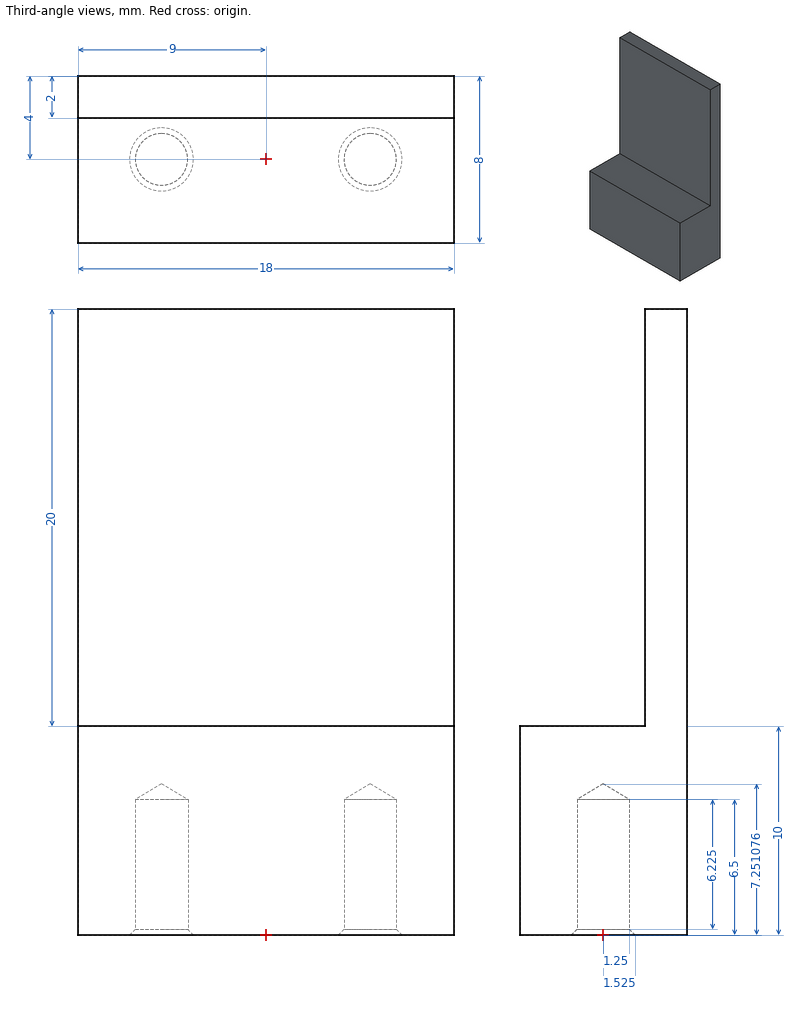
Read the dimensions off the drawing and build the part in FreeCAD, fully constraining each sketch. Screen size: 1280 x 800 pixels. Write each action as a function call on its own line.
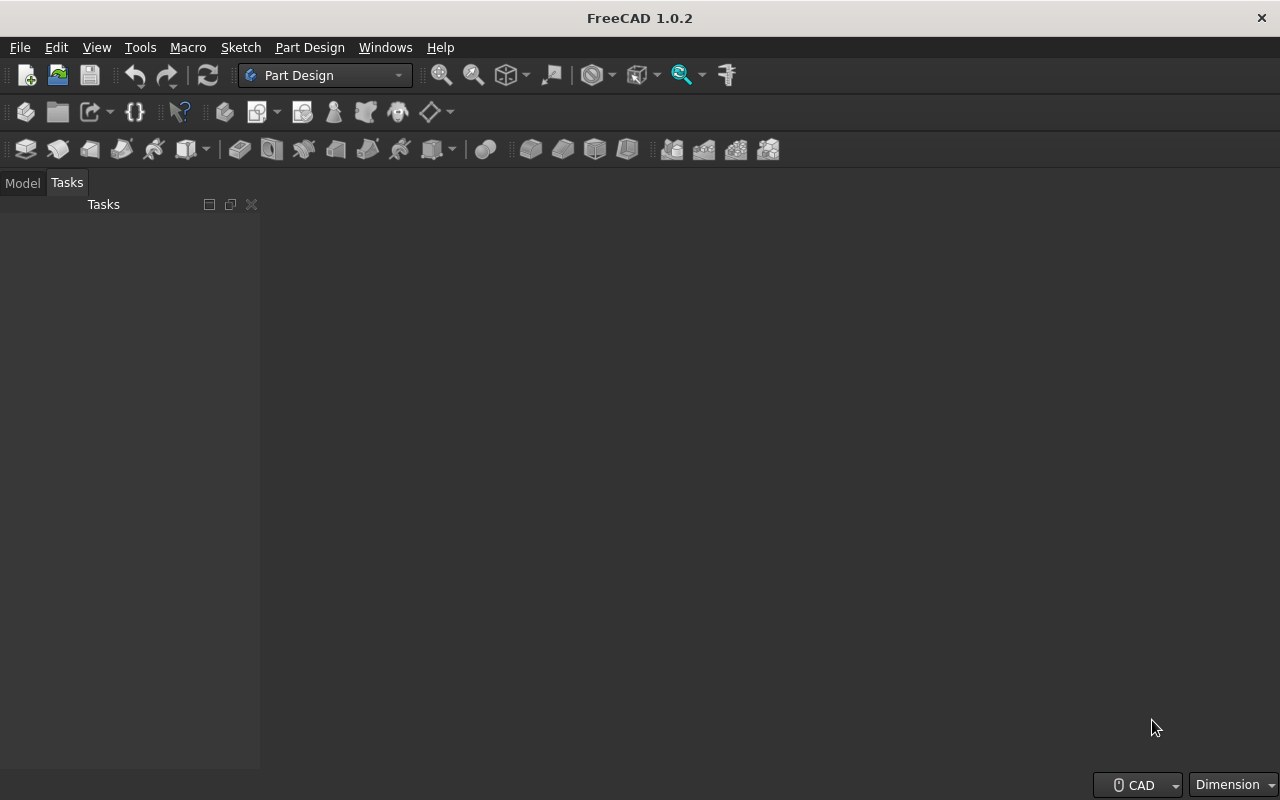
click(26, 76)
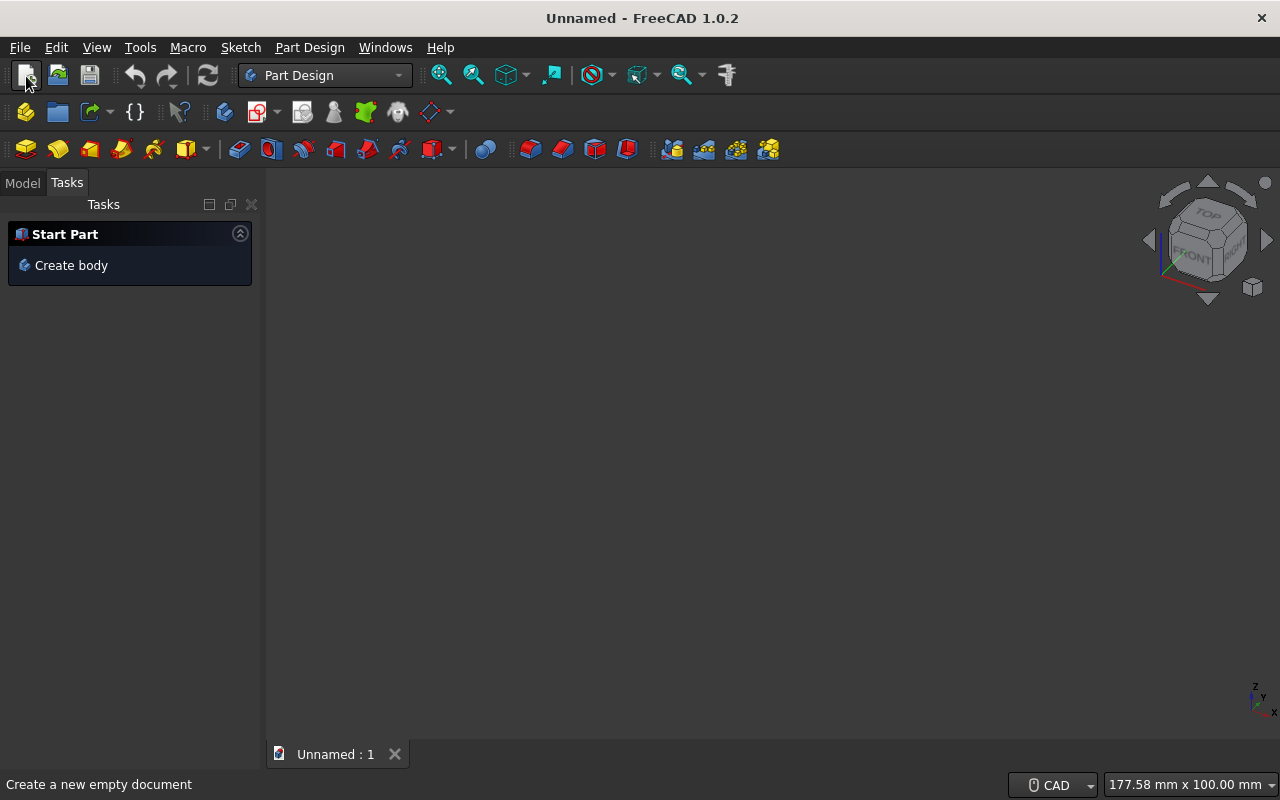
click(258, 112)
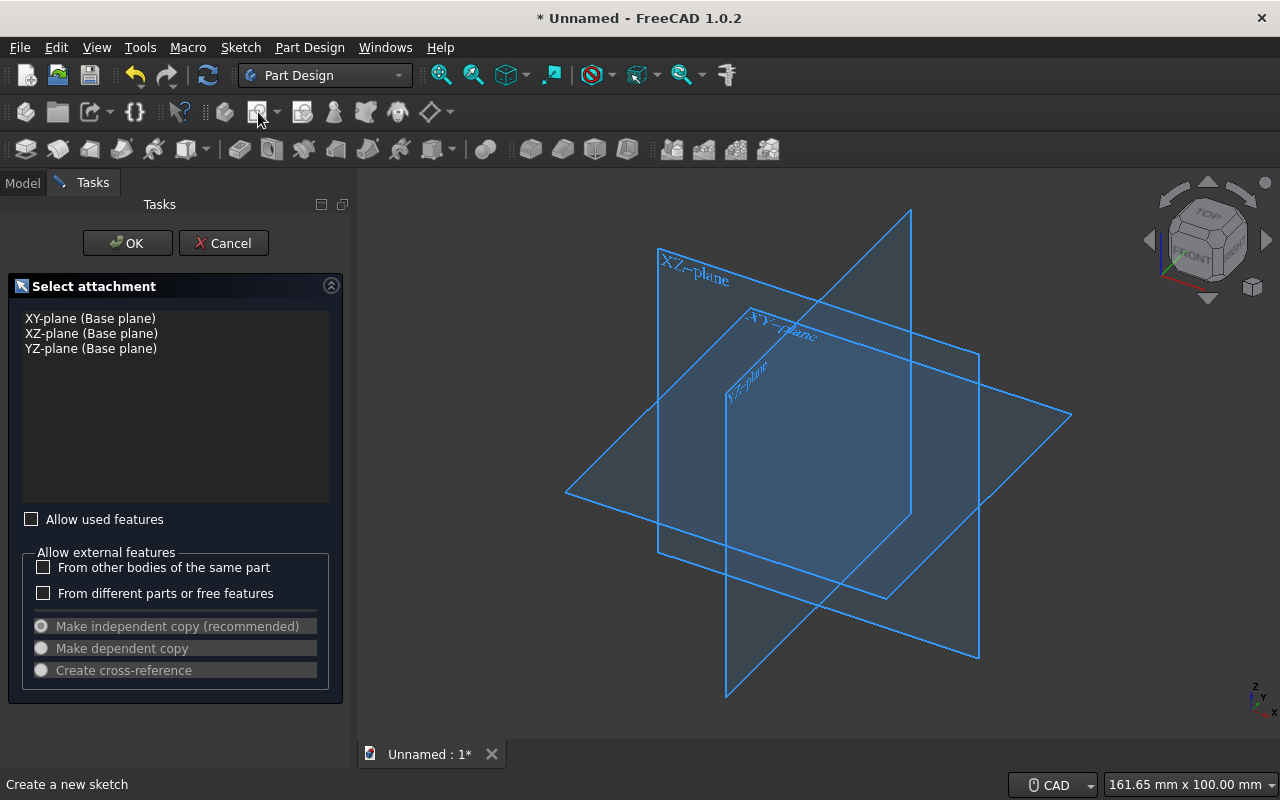
click(82, 318)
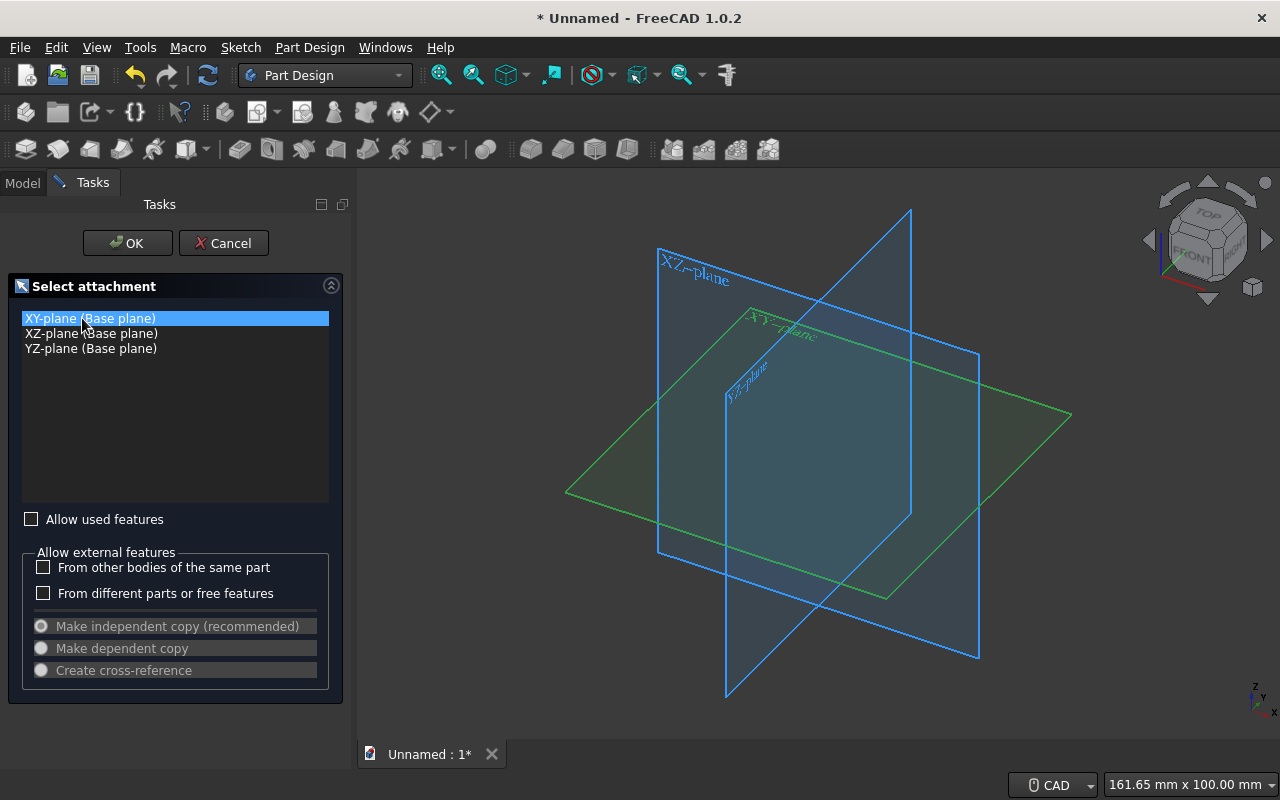
click(128, 243)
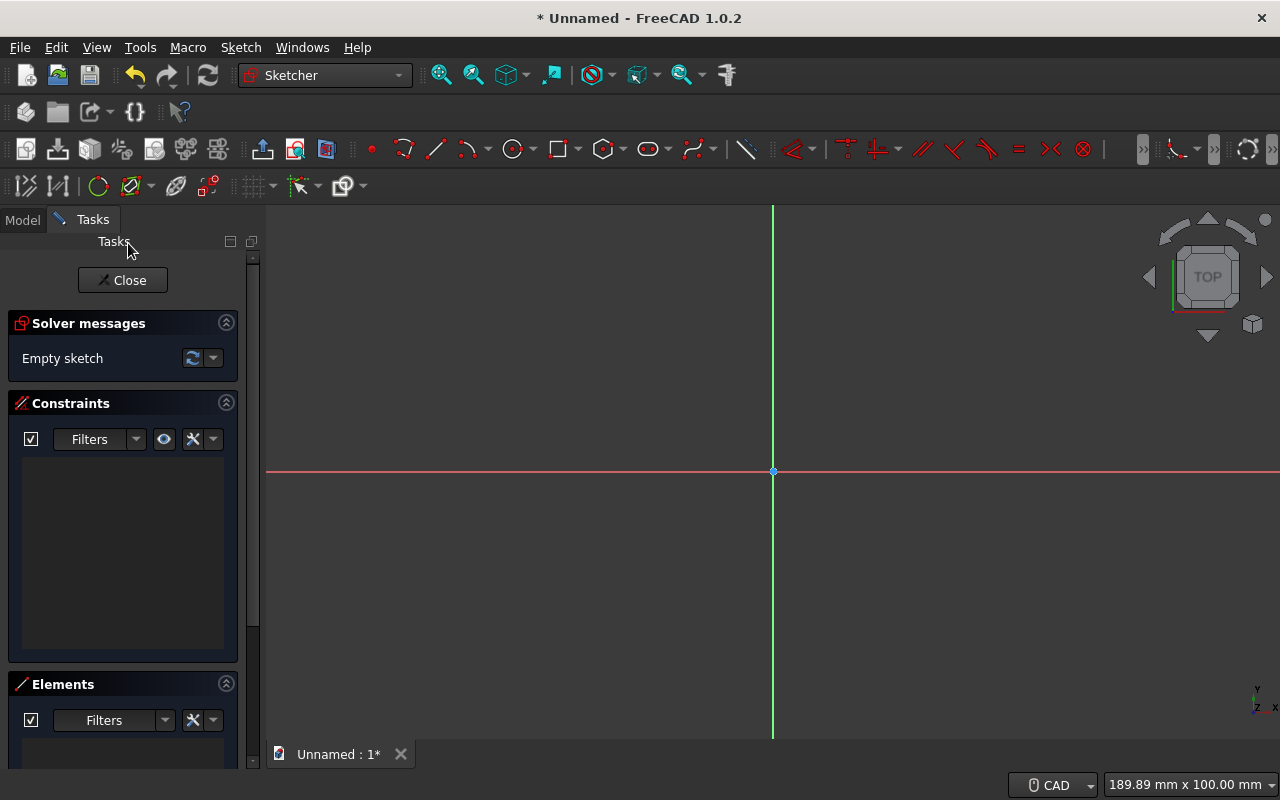
scroll(787, 472, up, 9)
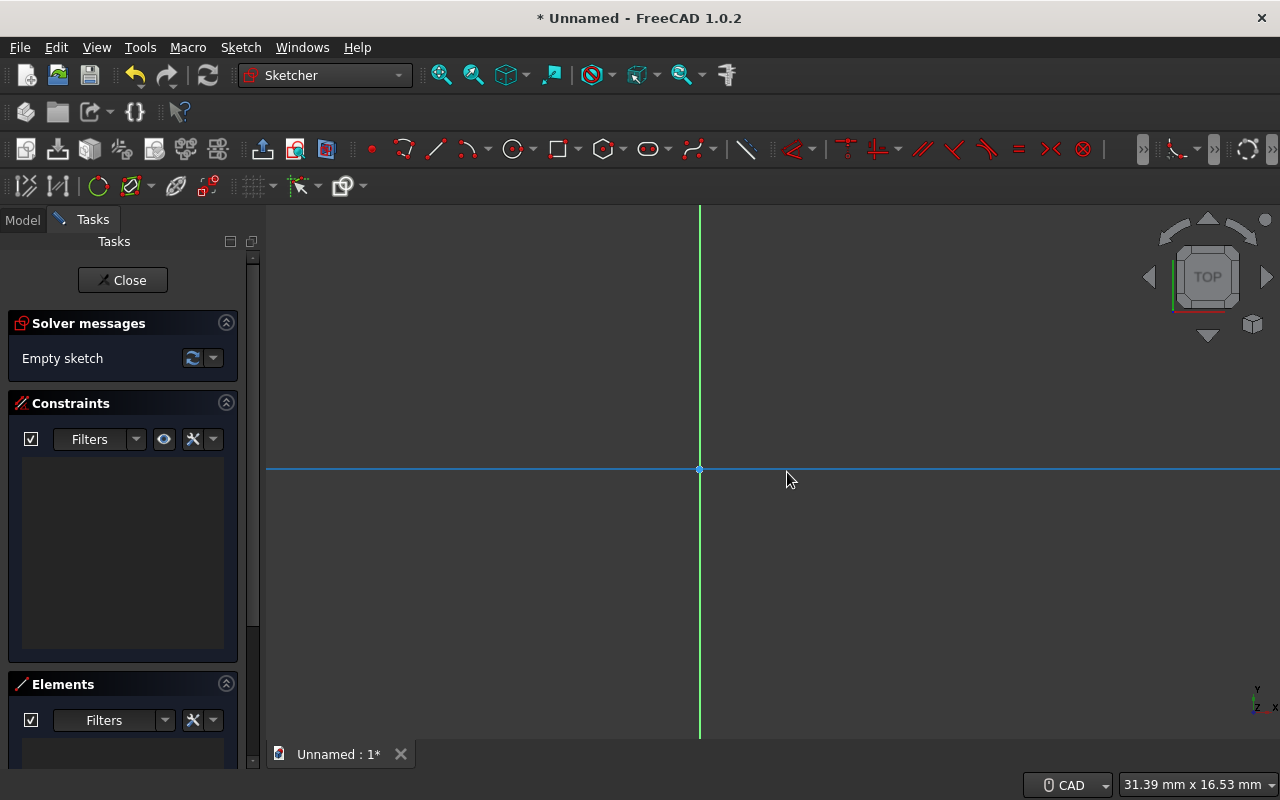
key(g)
key(v)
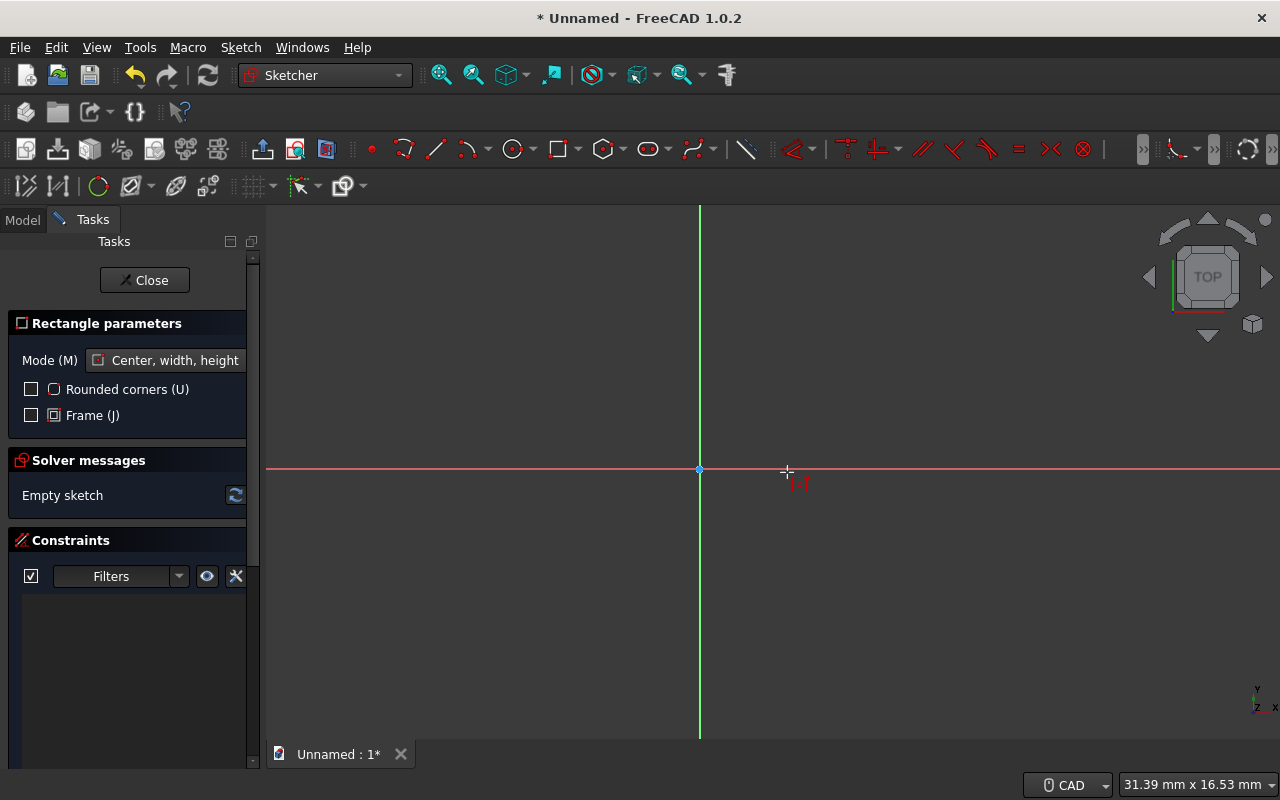
click(700, 469)
click(990, 340)
key(Escape)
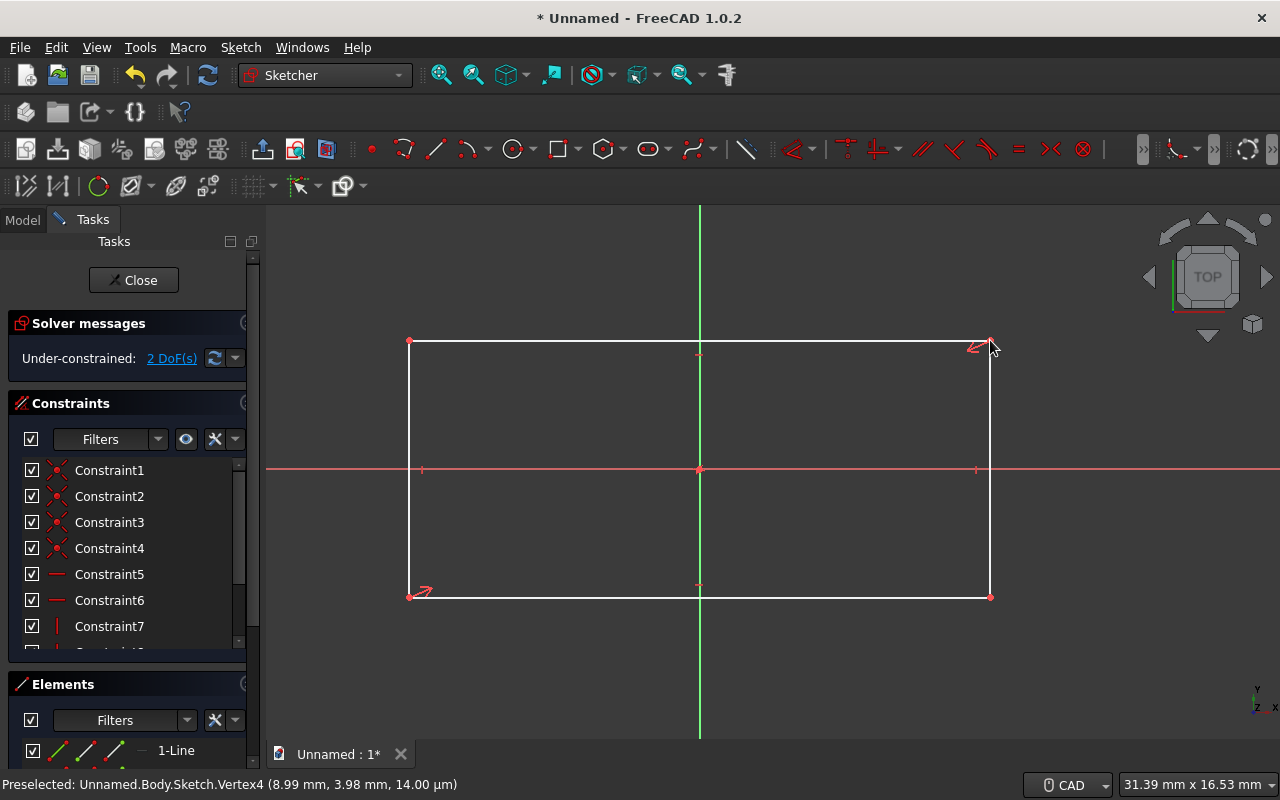
click(990, 521)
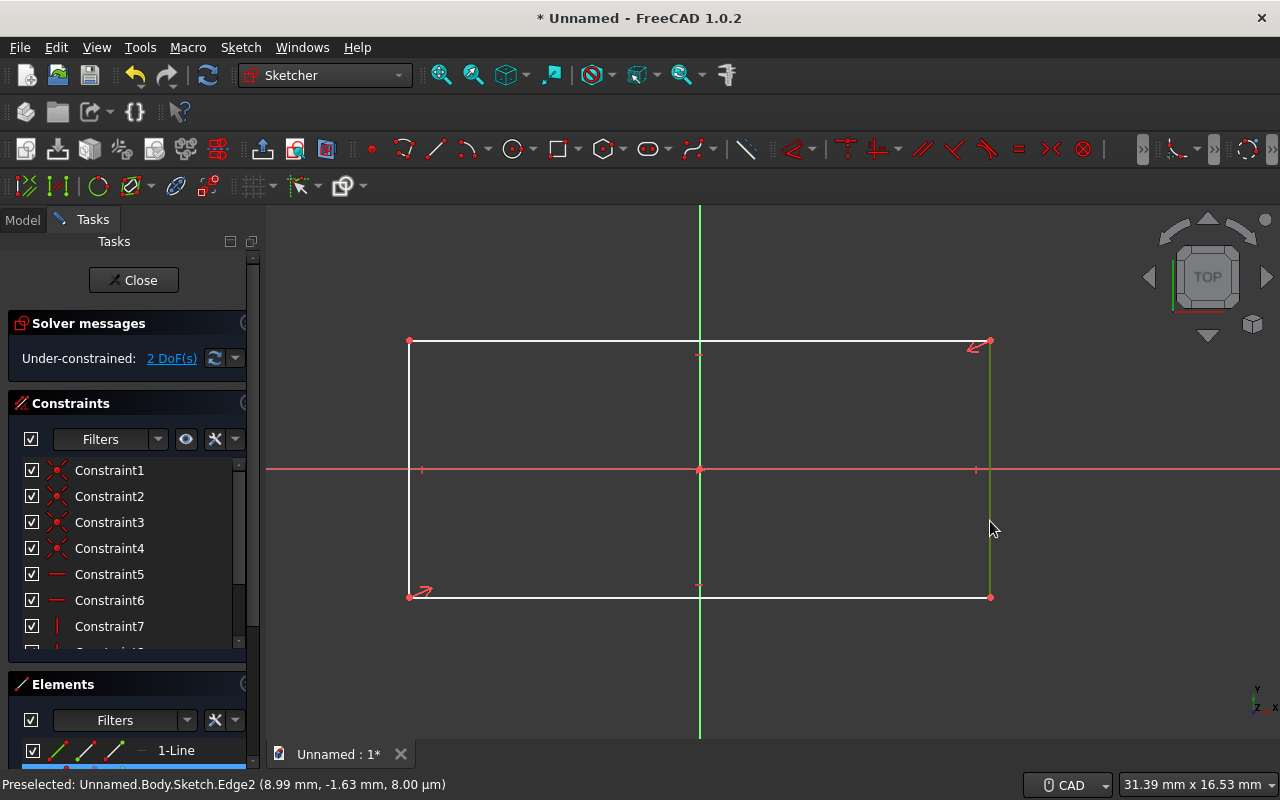
click(814, 150)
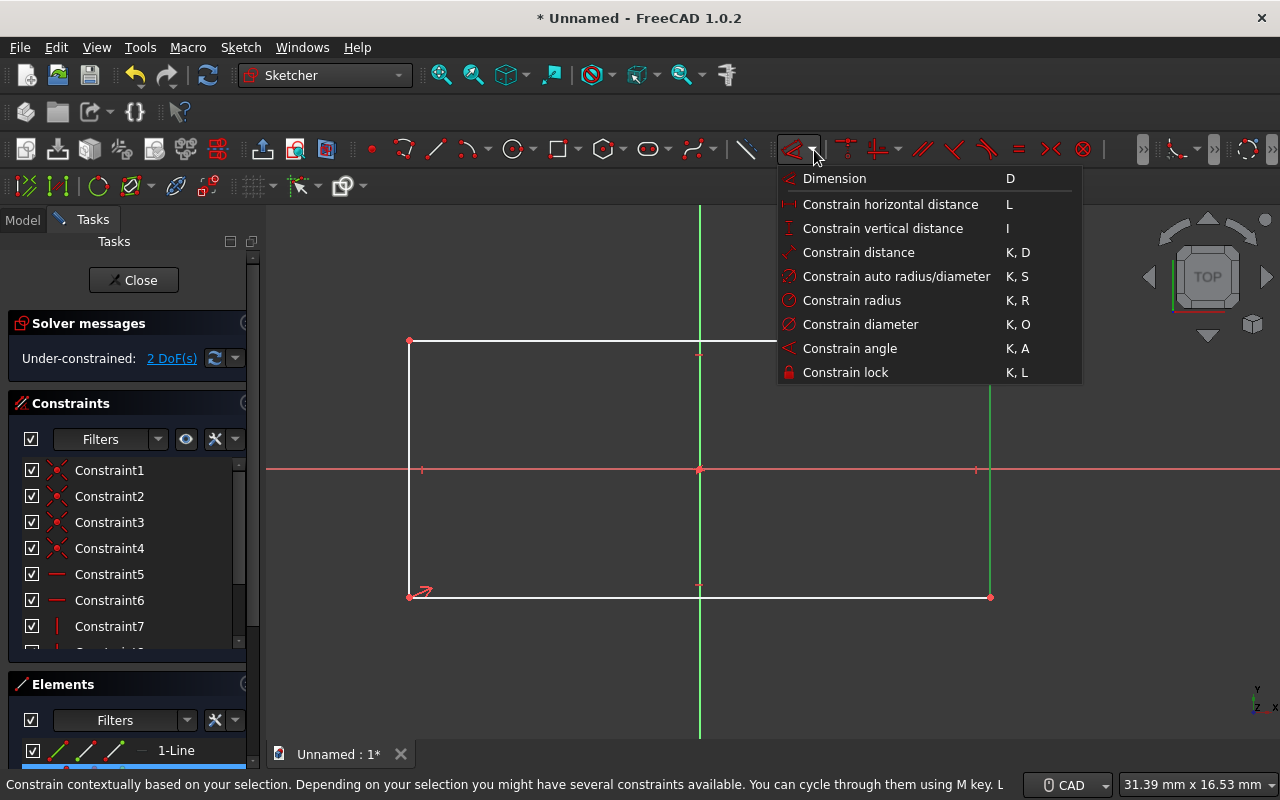
click(930, 228)